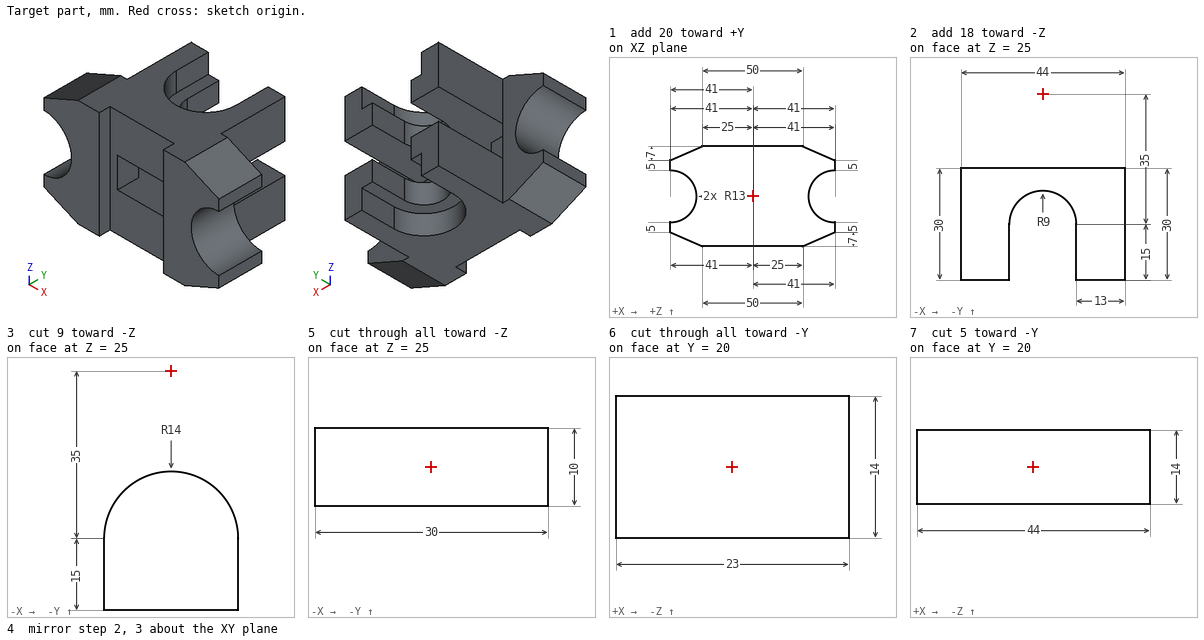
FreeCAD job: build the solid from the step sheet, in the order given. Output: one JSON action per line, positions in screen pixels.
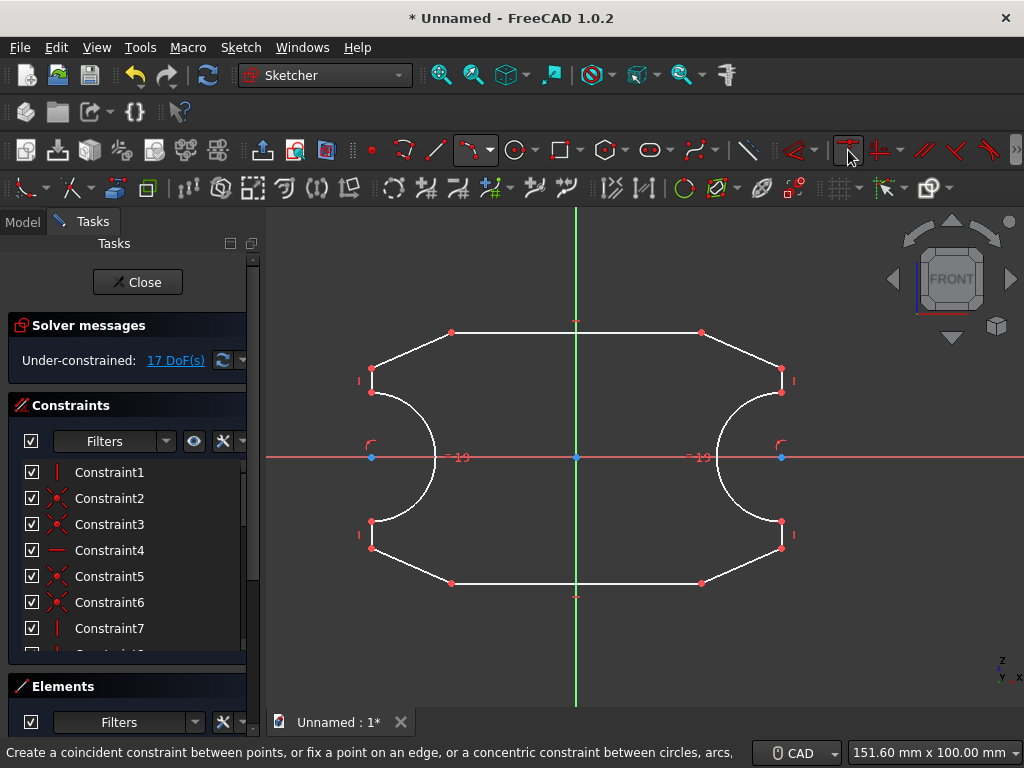
{"action": "left_click", "coordinate": [794, 150]}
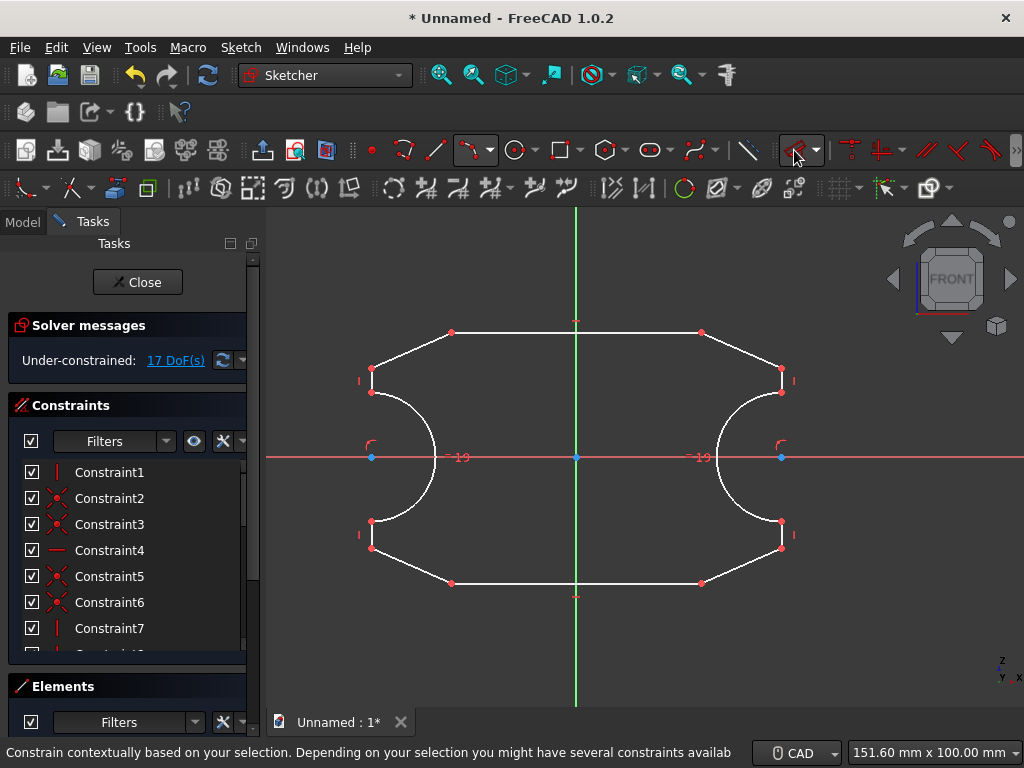
{"action": "left_click", "coordinate": [729, 419]}
{"action": "left_click", "coordinate": [703, 400]}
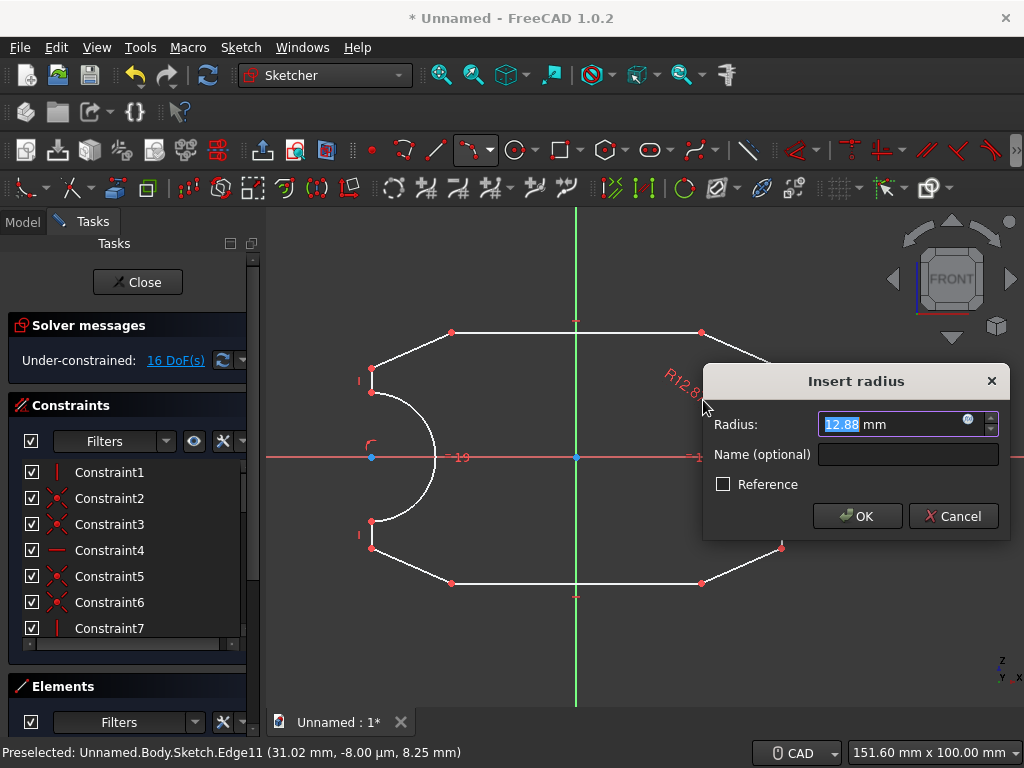
{"action": "type", "text": "13"}
{"action": "key", "text": "Return"}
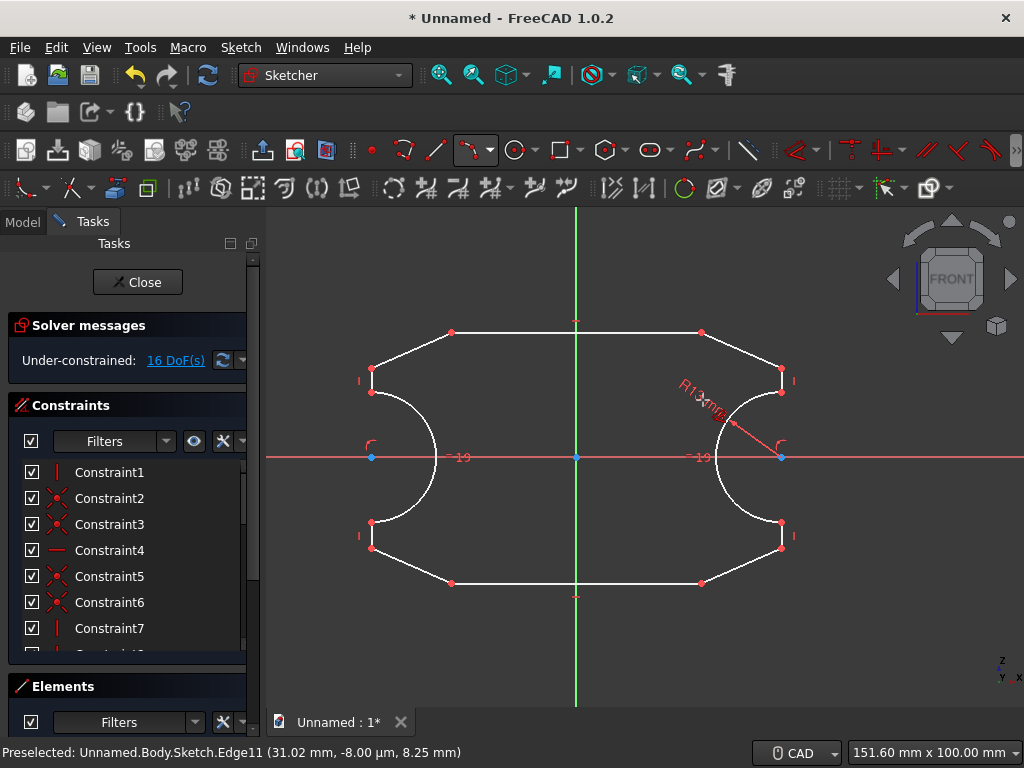
{"action": "scroll", "coordinate": [372, 383], "scroll_direction": "up", "scroll_amount": 3}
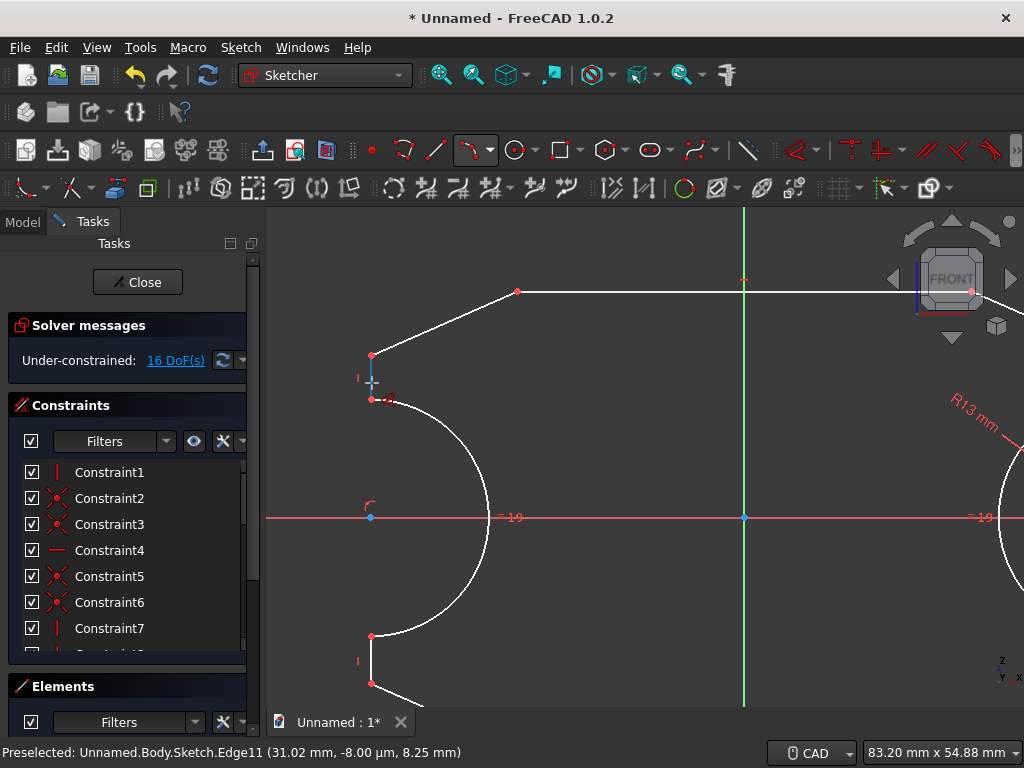
{"action": "left_click", "coordinate": [371, 382]}
{"action": "left_click", "coordinate": [337, 378]}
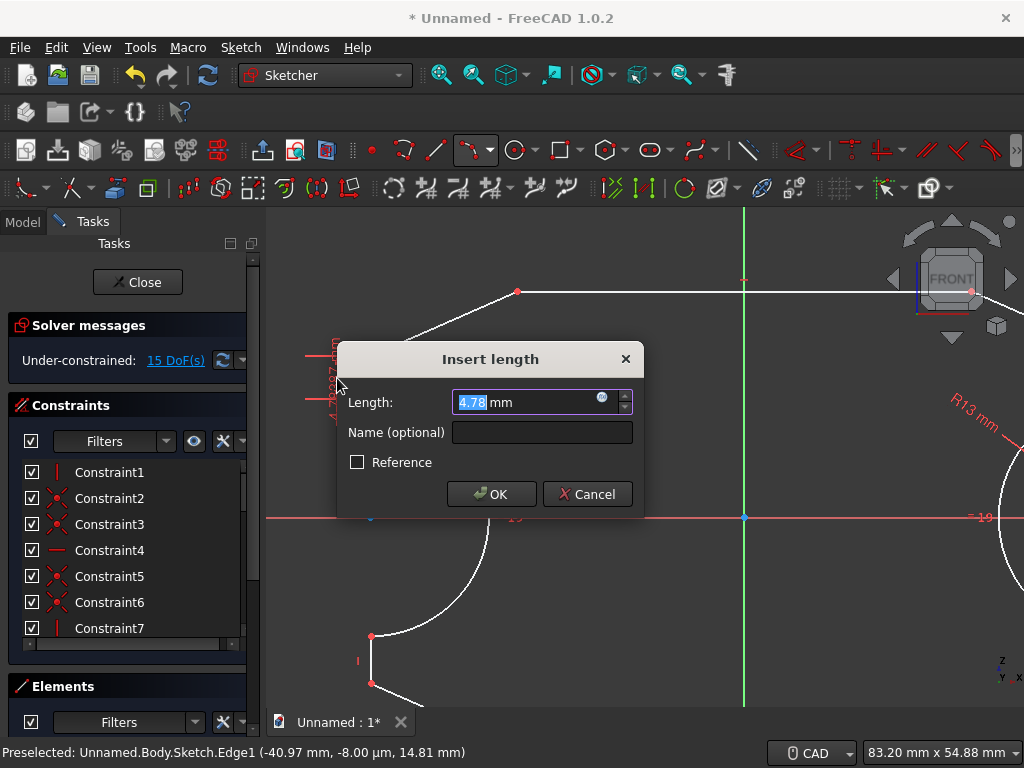
{"action": "type", "text": "5"}
{"action": "key", "text": "Return"}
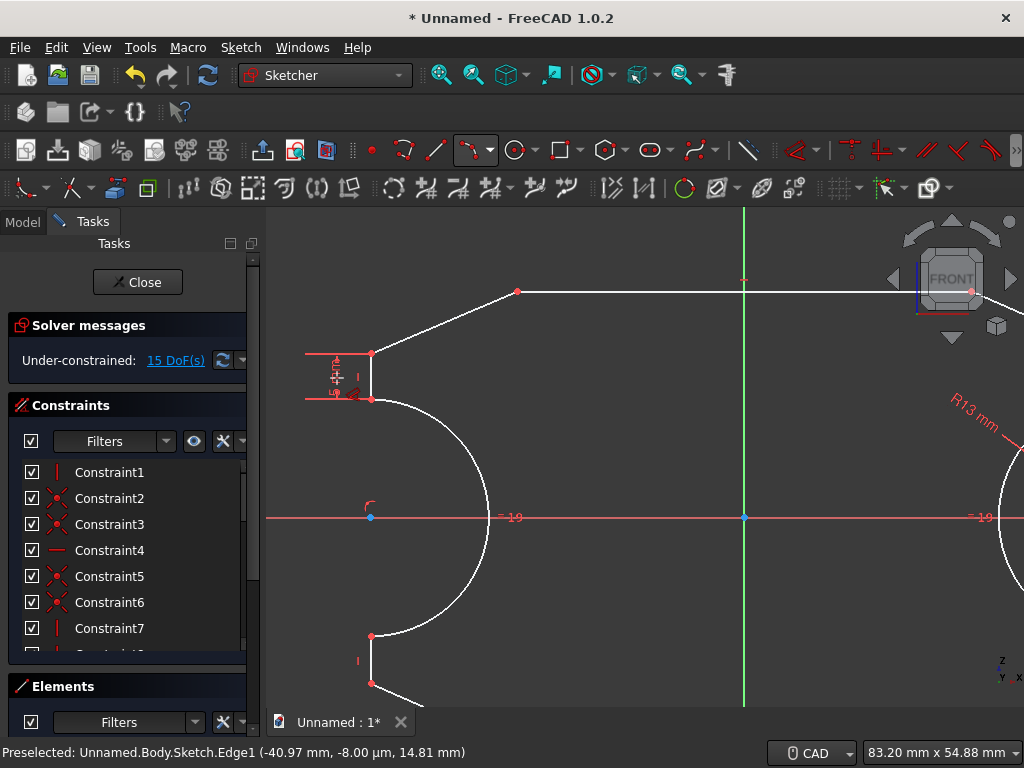
{"action": "scroll", "coordinate": [372, 383], "scroll_direction": "down", "scroll_amount": 3}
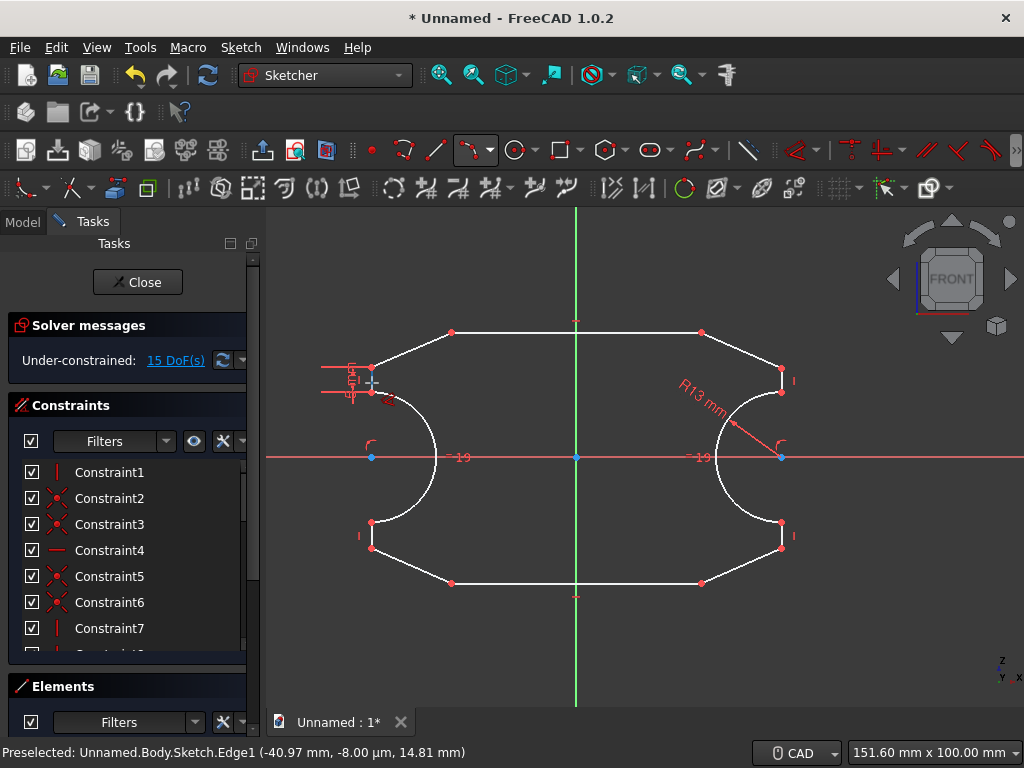
{"action": "scroll", "coordinate": [782, 375], "scroll_direction": "up", "scroll_amount": 4}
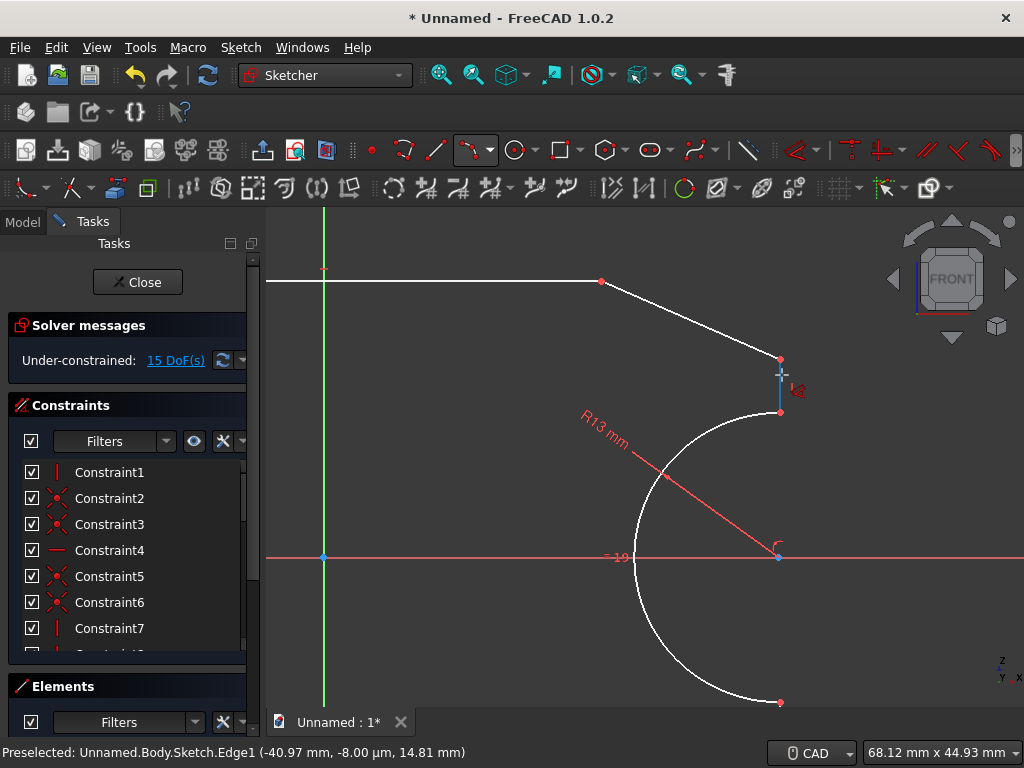
{"action": "left_click", "coordinate": [780, 376]}
{"action": "left_click", "coordinate": [814, 386]}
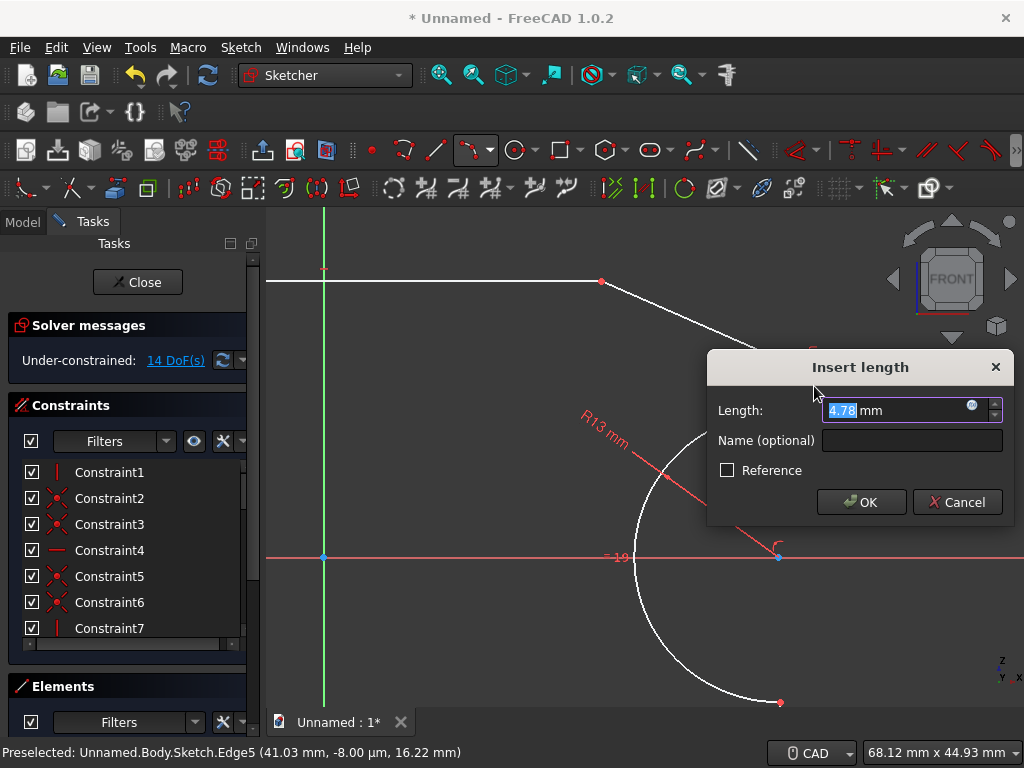
{"action": "type", "text": "5"}
{"action": "key", "text": "Return"}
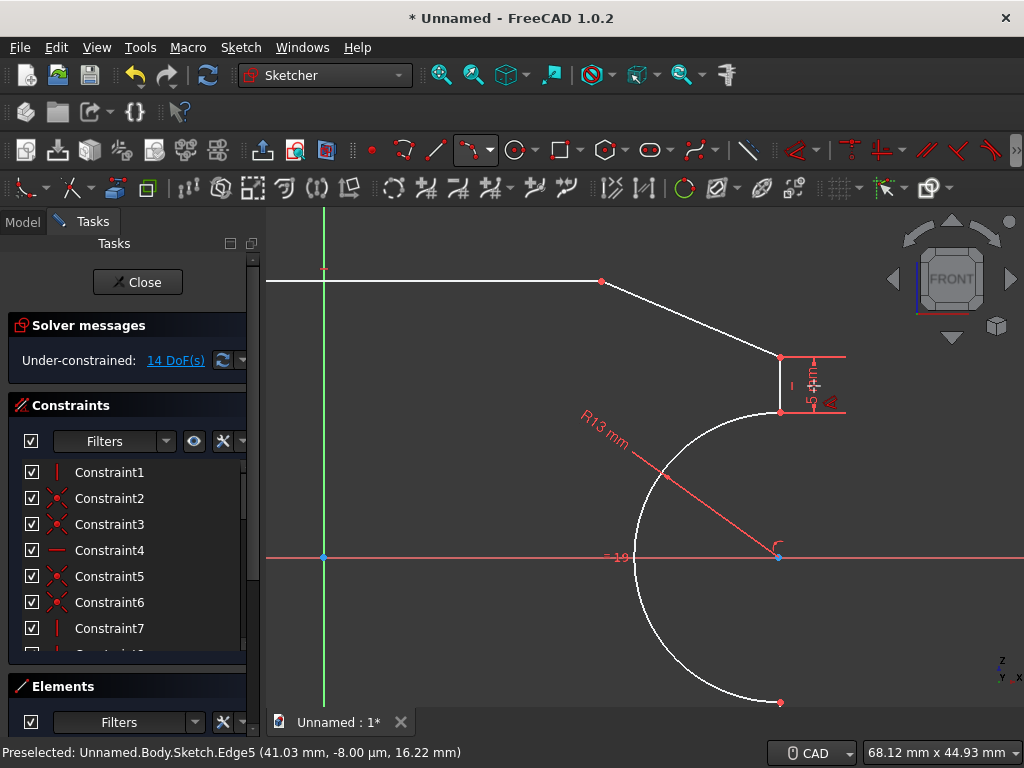
{"action": "scroll", "coordinate": [783, 375], "scroll_direction": "down", "scroll_amount": 4}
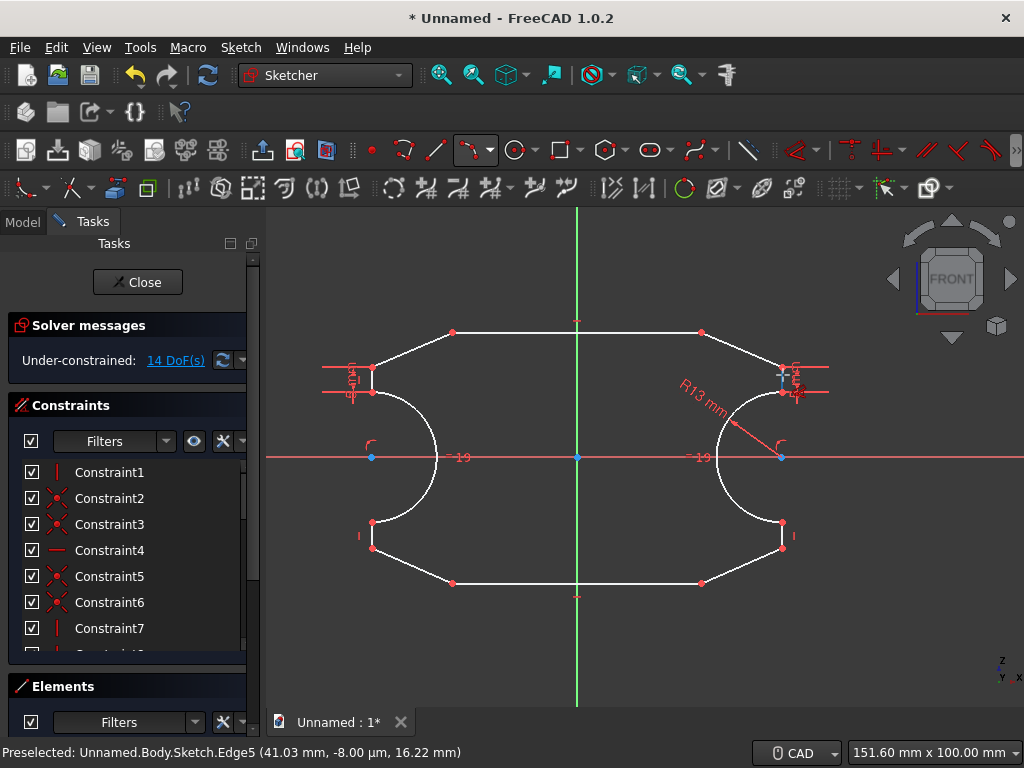
{"action": "scroll", "coordinate": [782, 530], "scroll_direction": "up", "scroll_amount": 3}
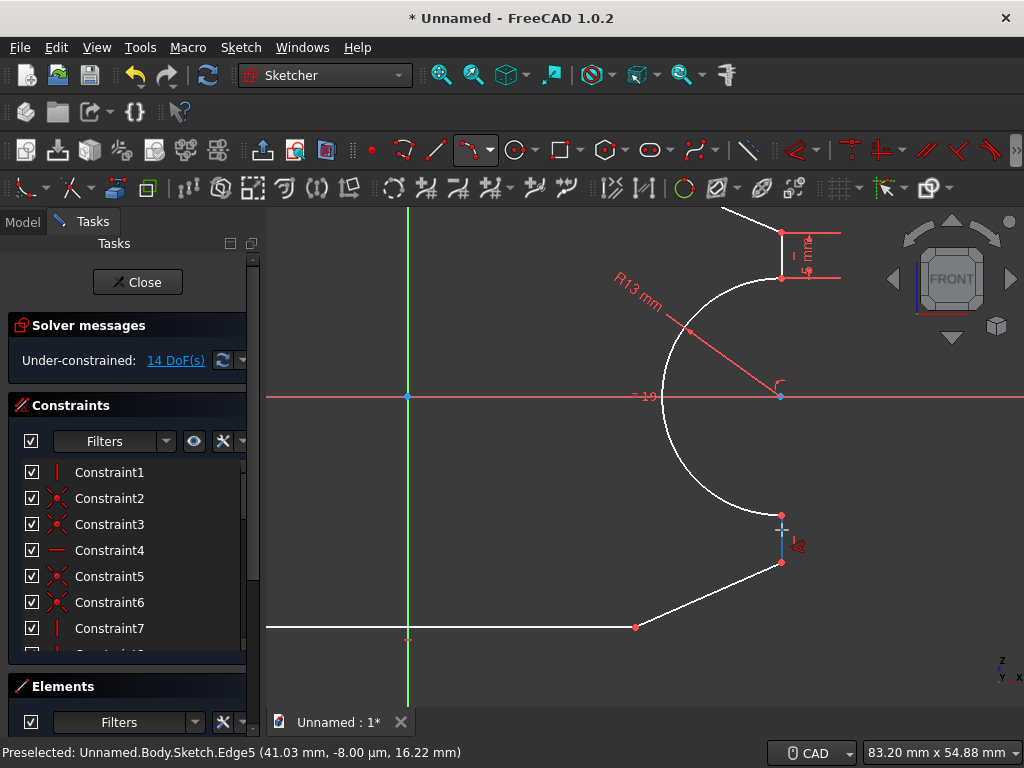
{"action": "left_click", "coordinate": [782, 530]}
{"action": "left_click", "coordinate": [816, 539]}